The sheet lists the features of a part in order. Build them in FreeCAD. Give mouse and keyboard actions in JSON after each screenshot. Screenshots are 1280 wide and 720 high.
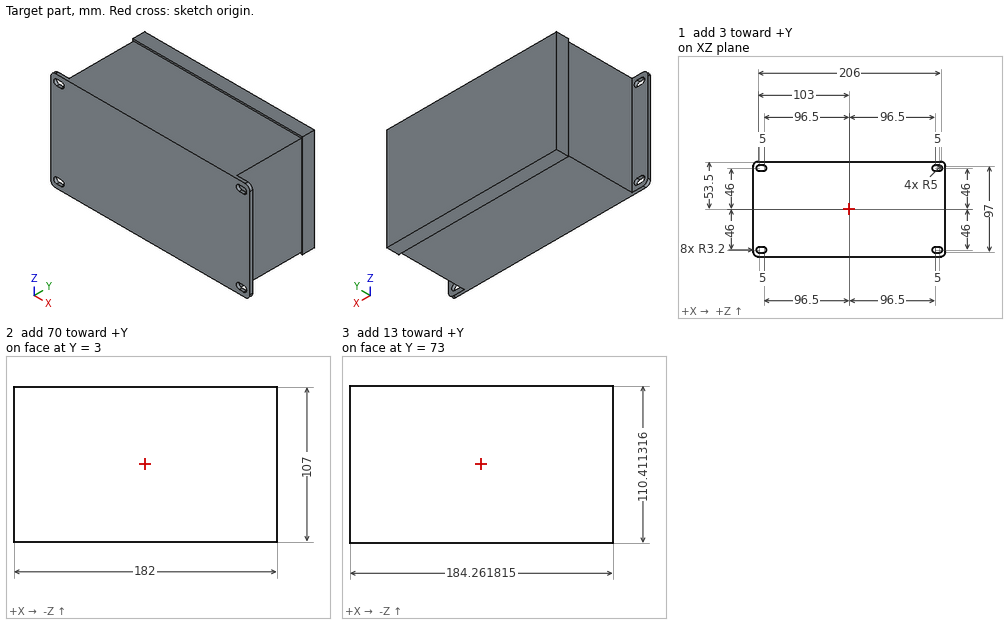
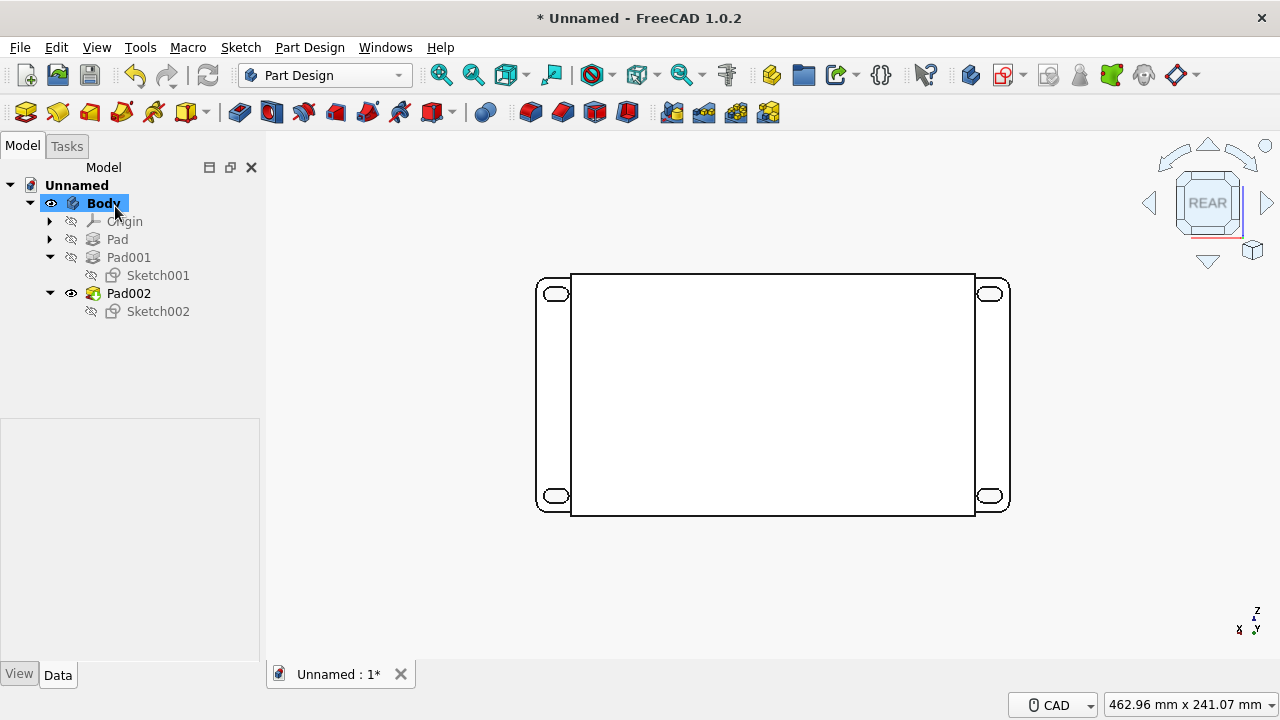
{"action": "key", "text": "0"}